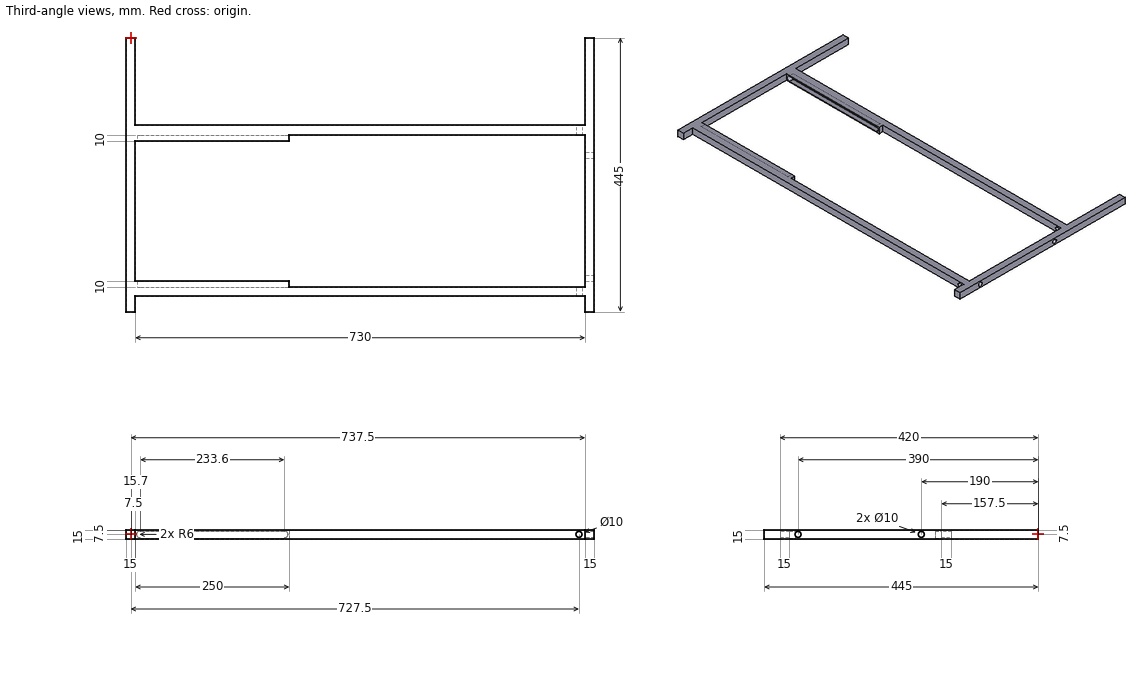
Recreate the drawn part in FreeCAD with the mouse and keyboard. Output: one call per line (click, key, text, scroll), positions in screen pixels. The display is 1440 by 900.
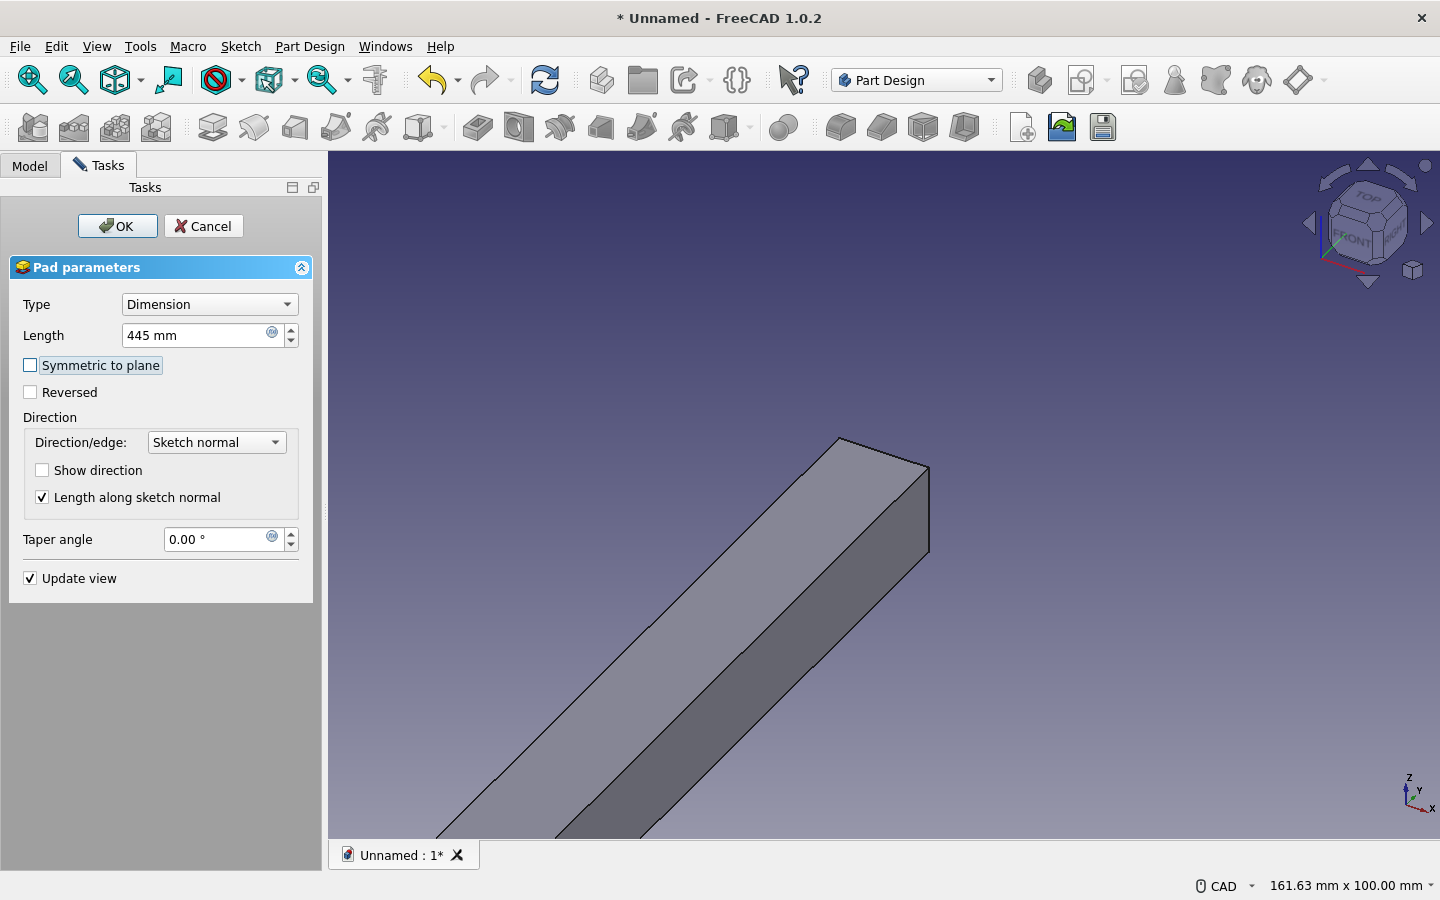
click(118, 226)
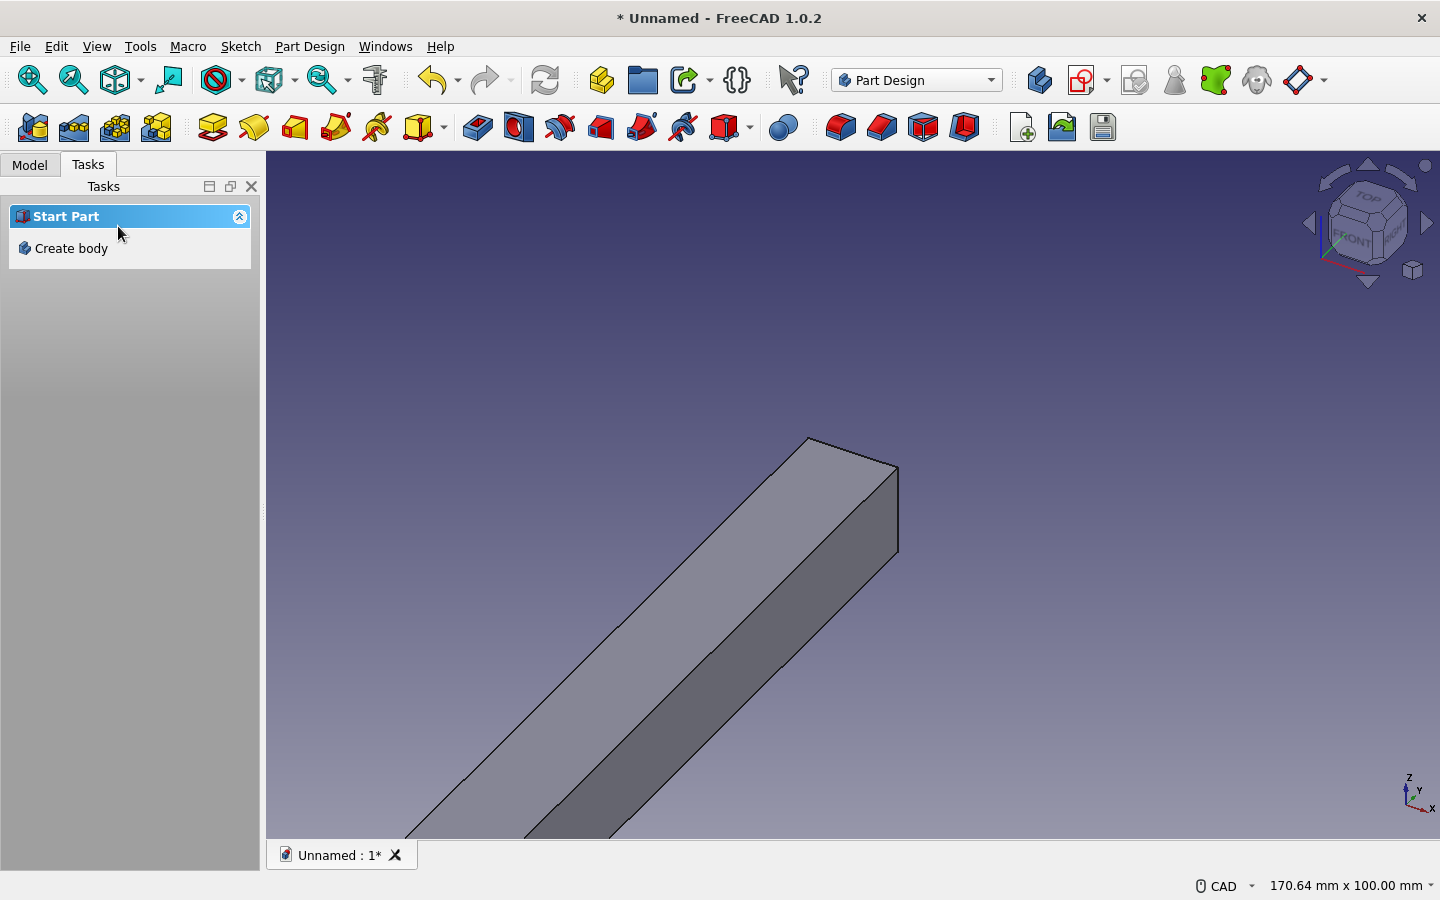
click(33, 80)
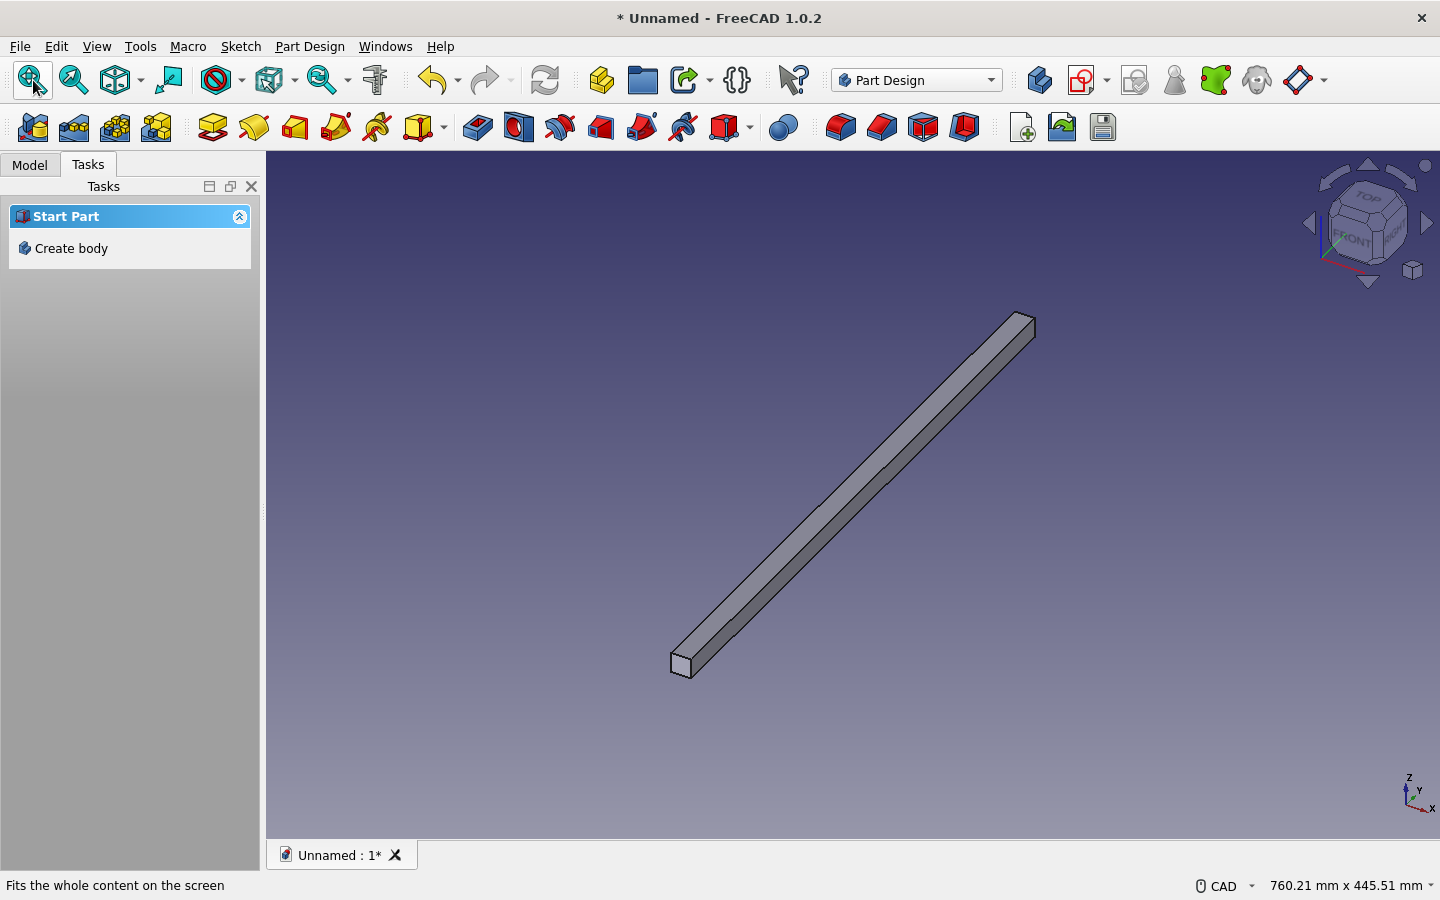
click(1040, 80)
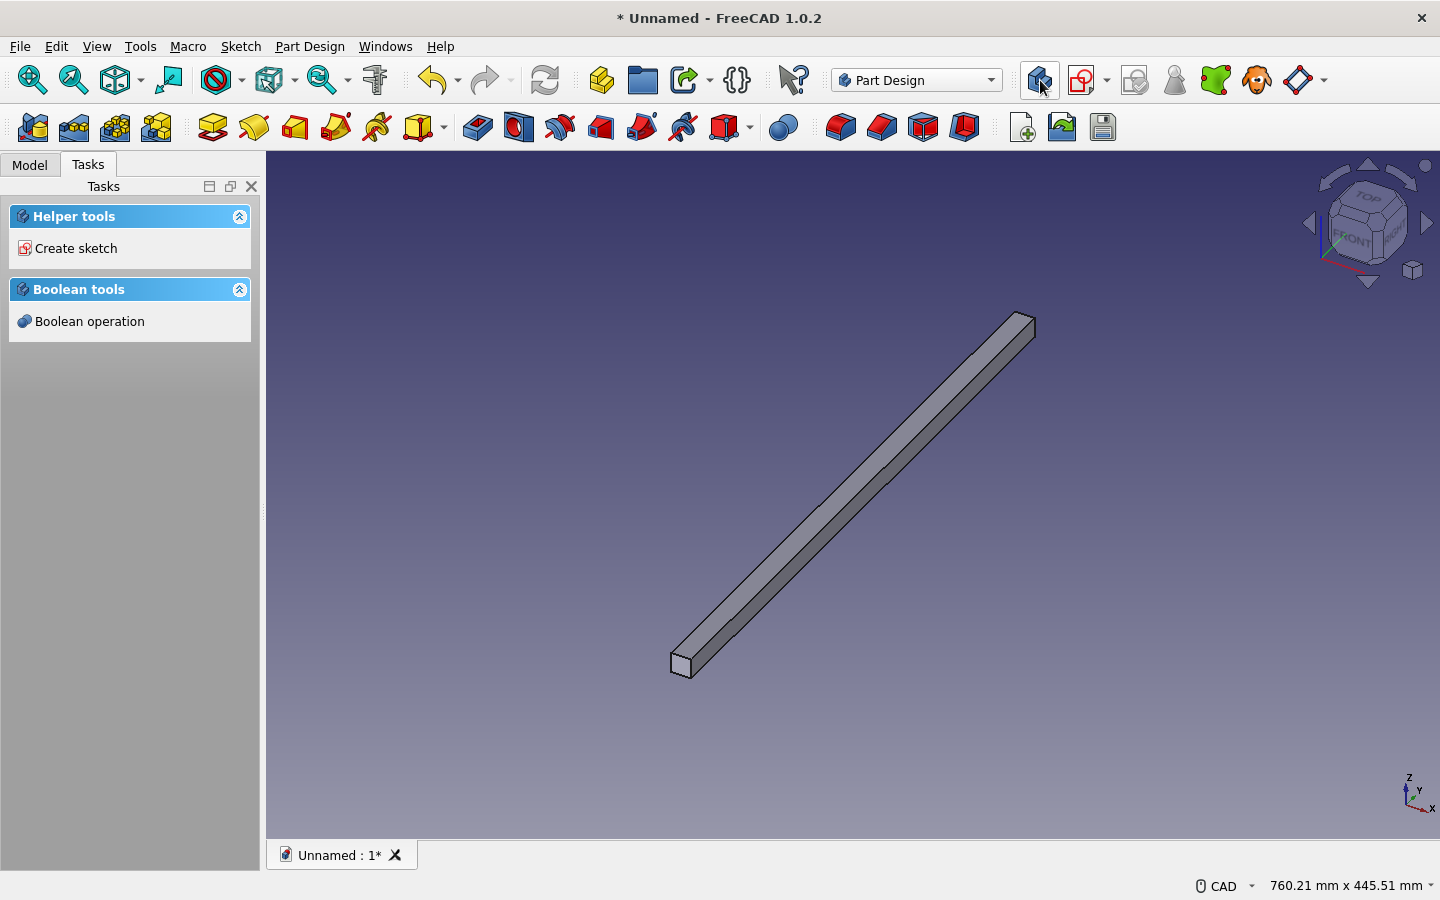
click(306, 799)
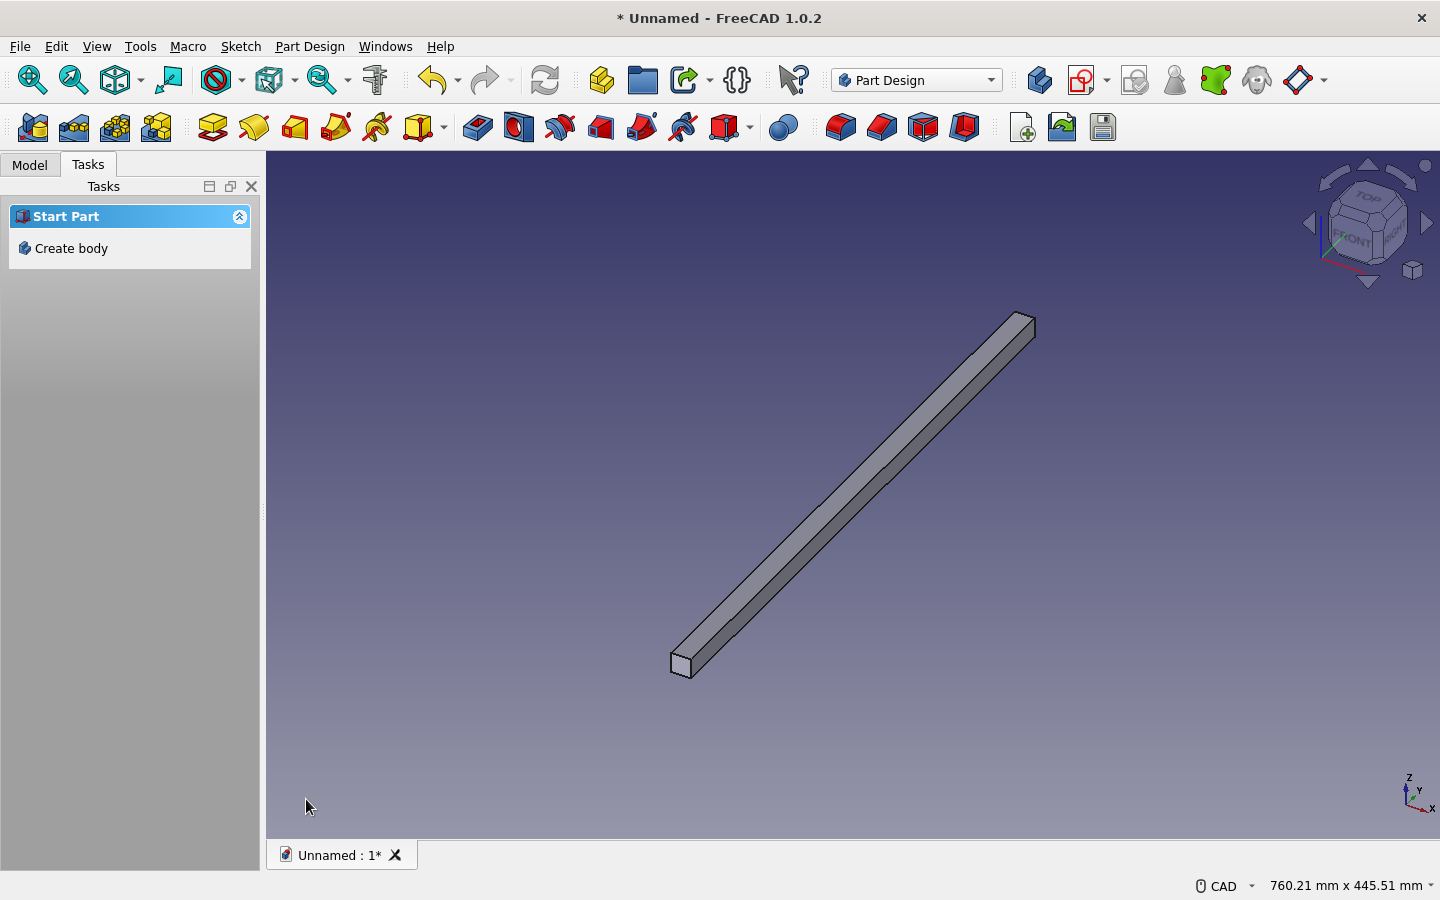
click(1080, 80)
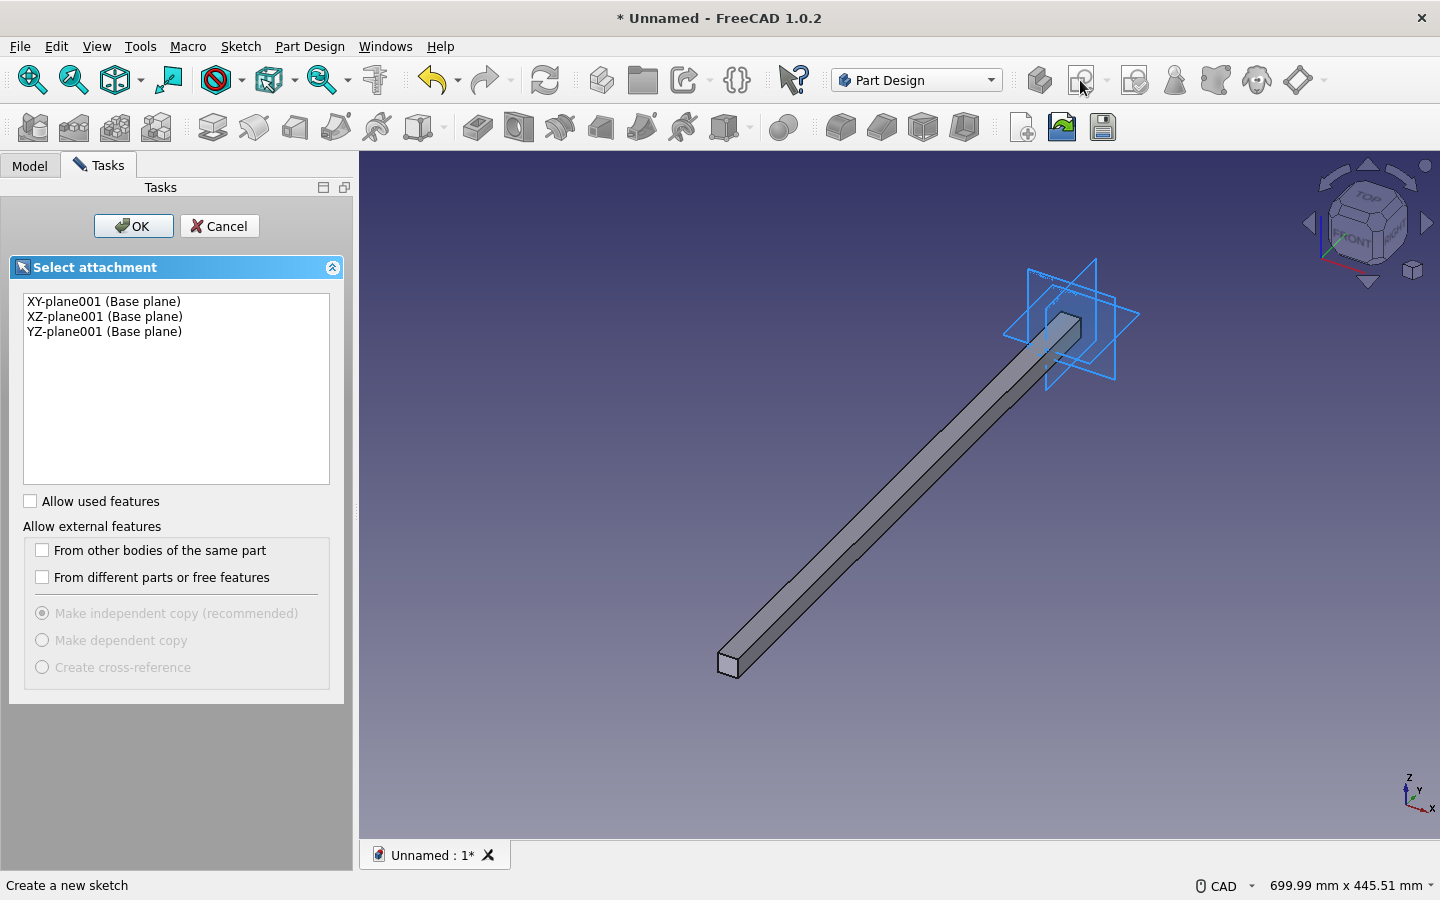
click(84, 316)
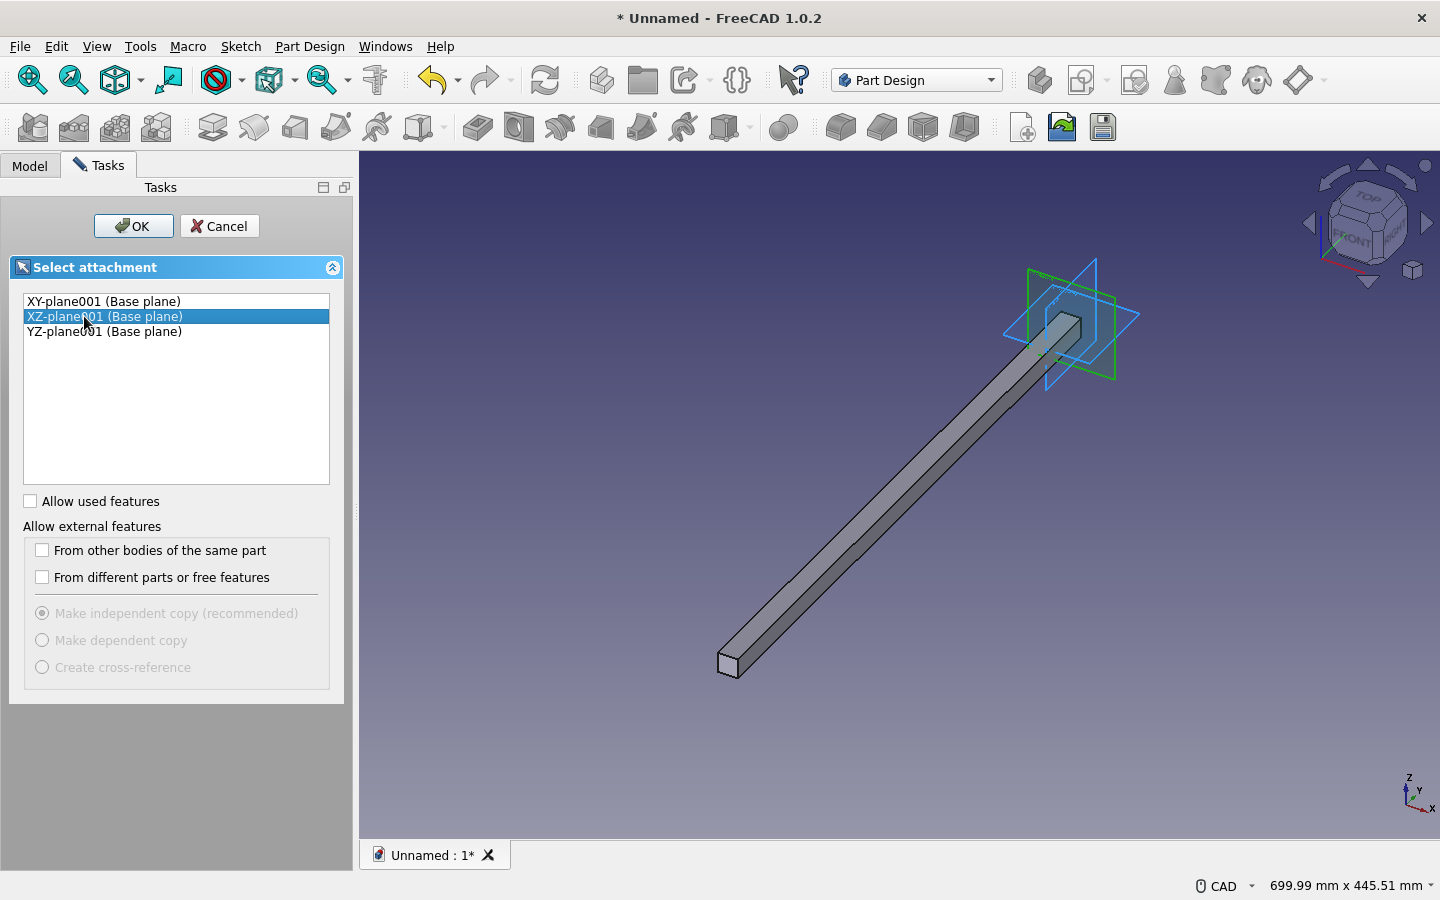
click(134, 226)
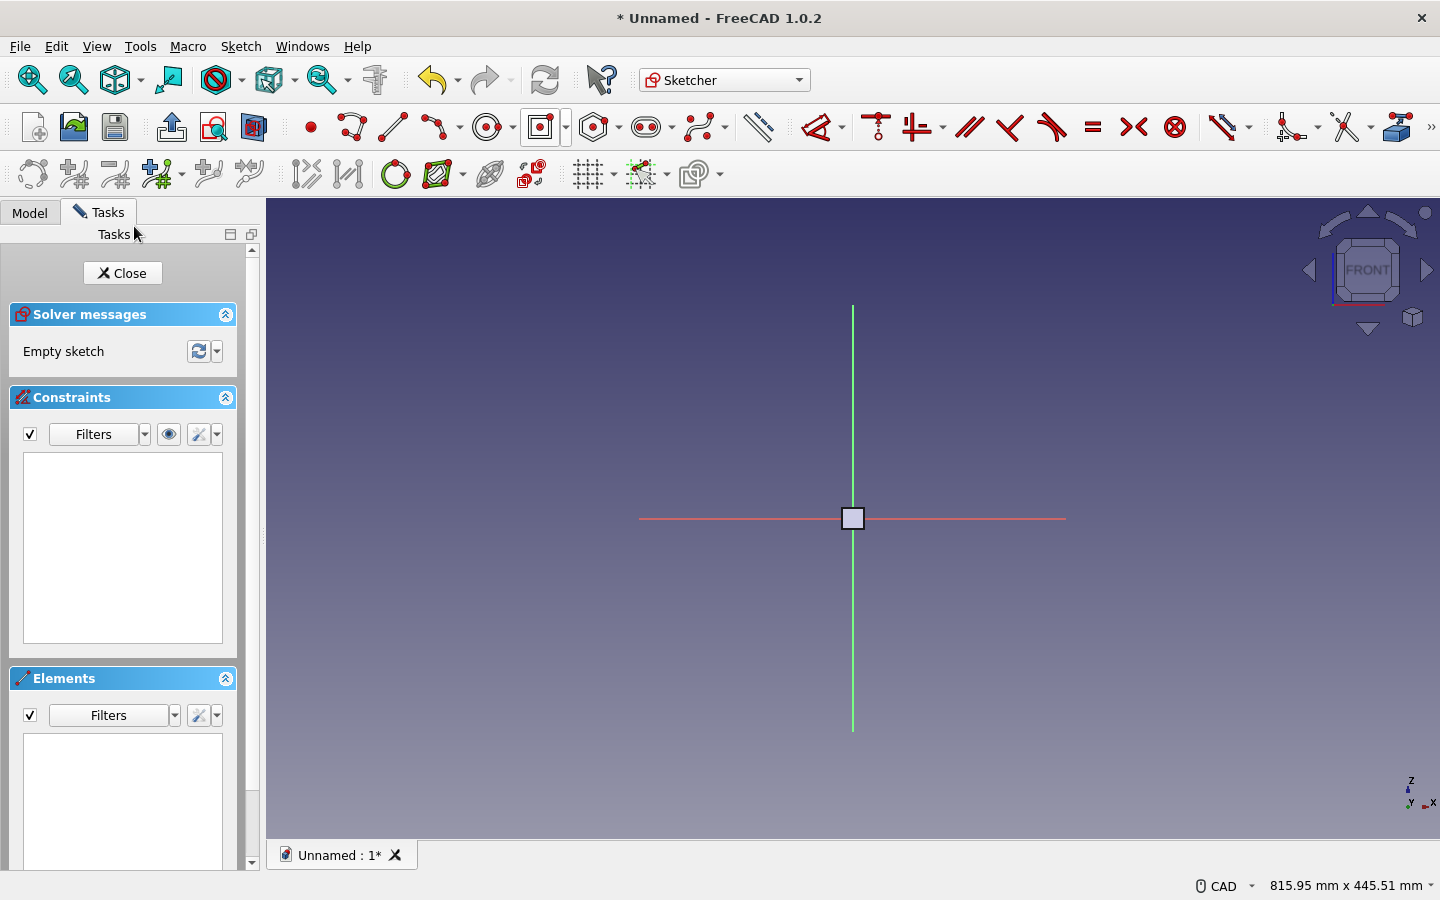
scroll(784, 518, down, 5)